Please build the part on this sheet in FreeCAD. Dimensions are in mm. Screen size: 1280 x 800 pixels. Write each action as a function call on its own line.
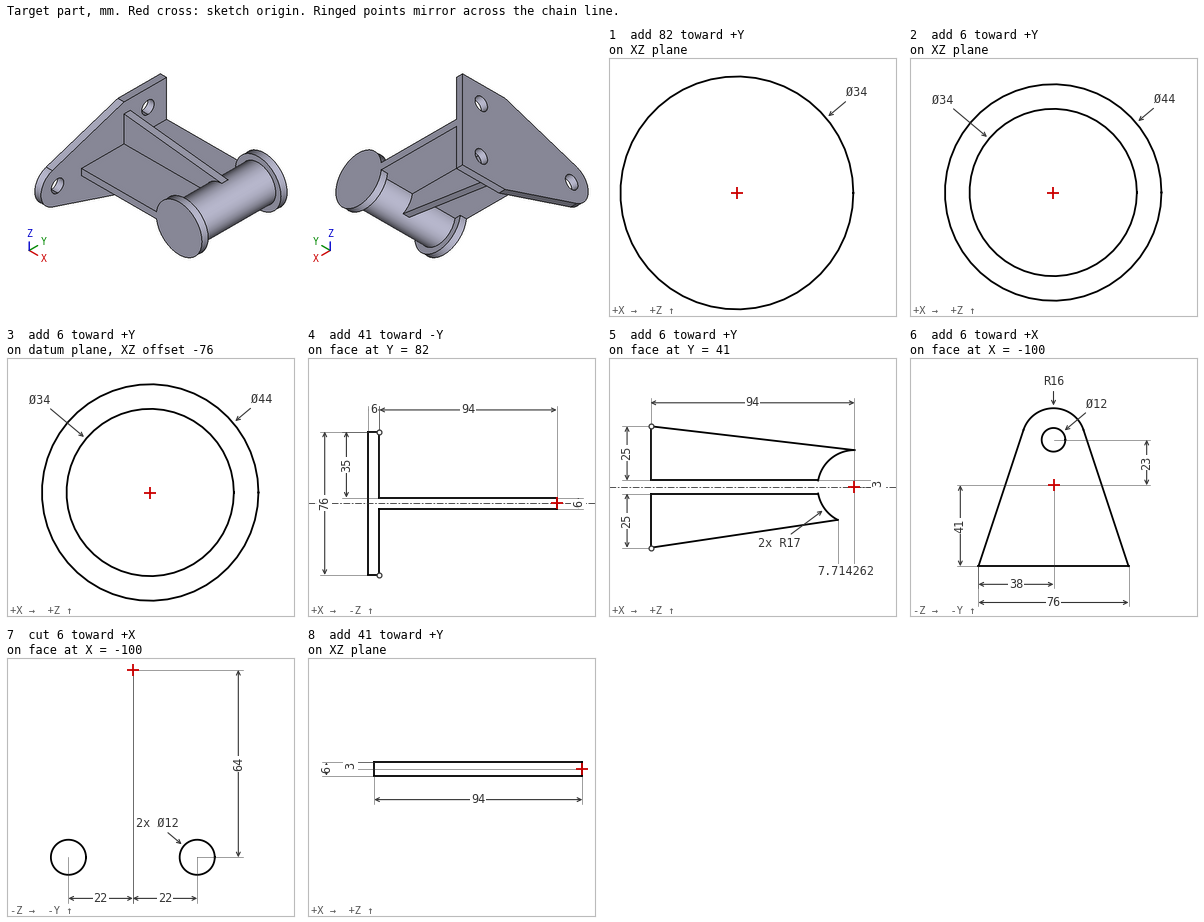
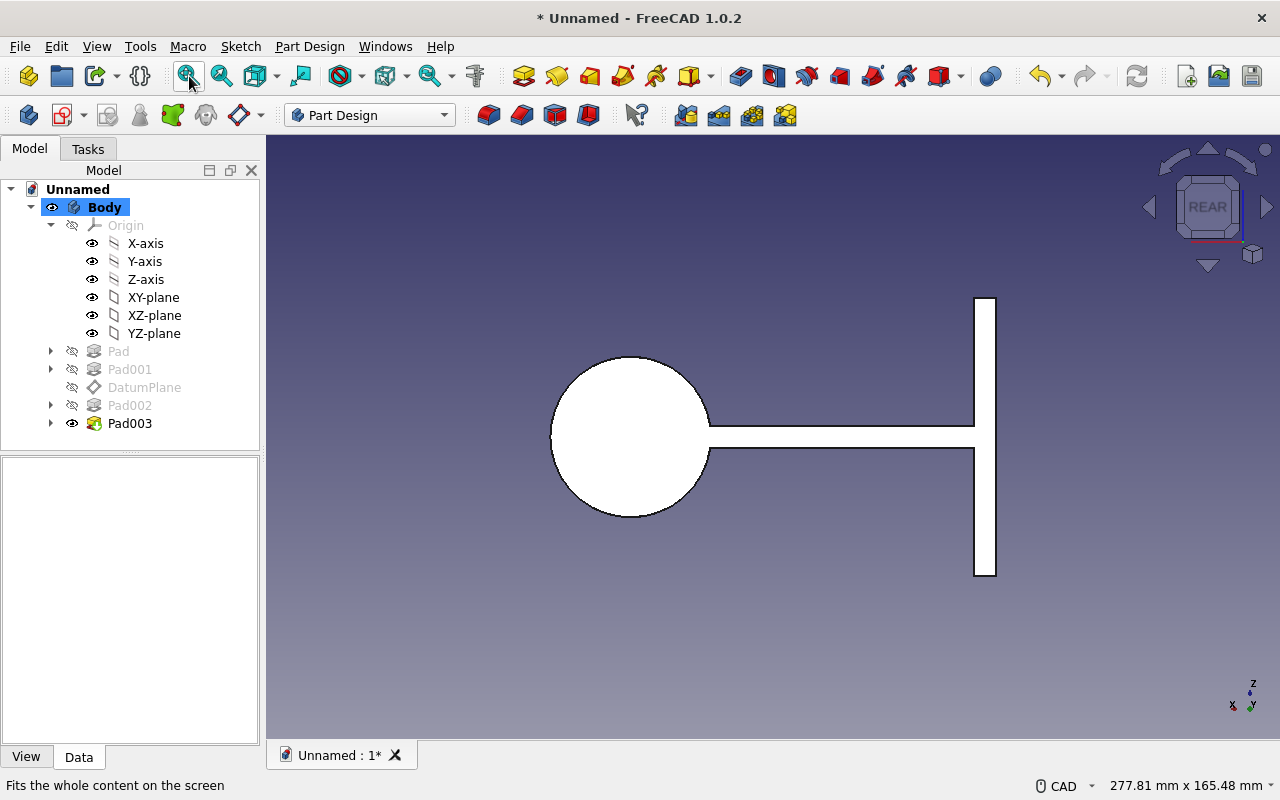
key(0)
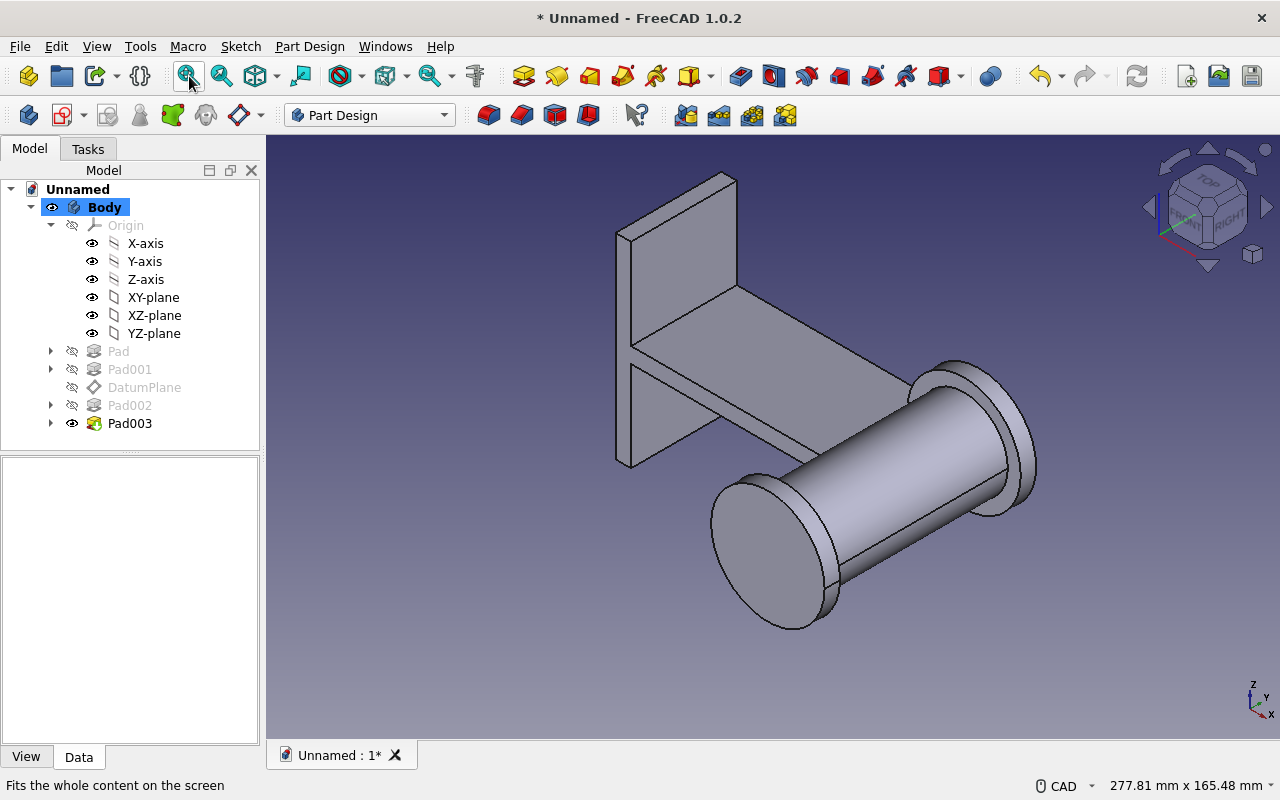
key(1)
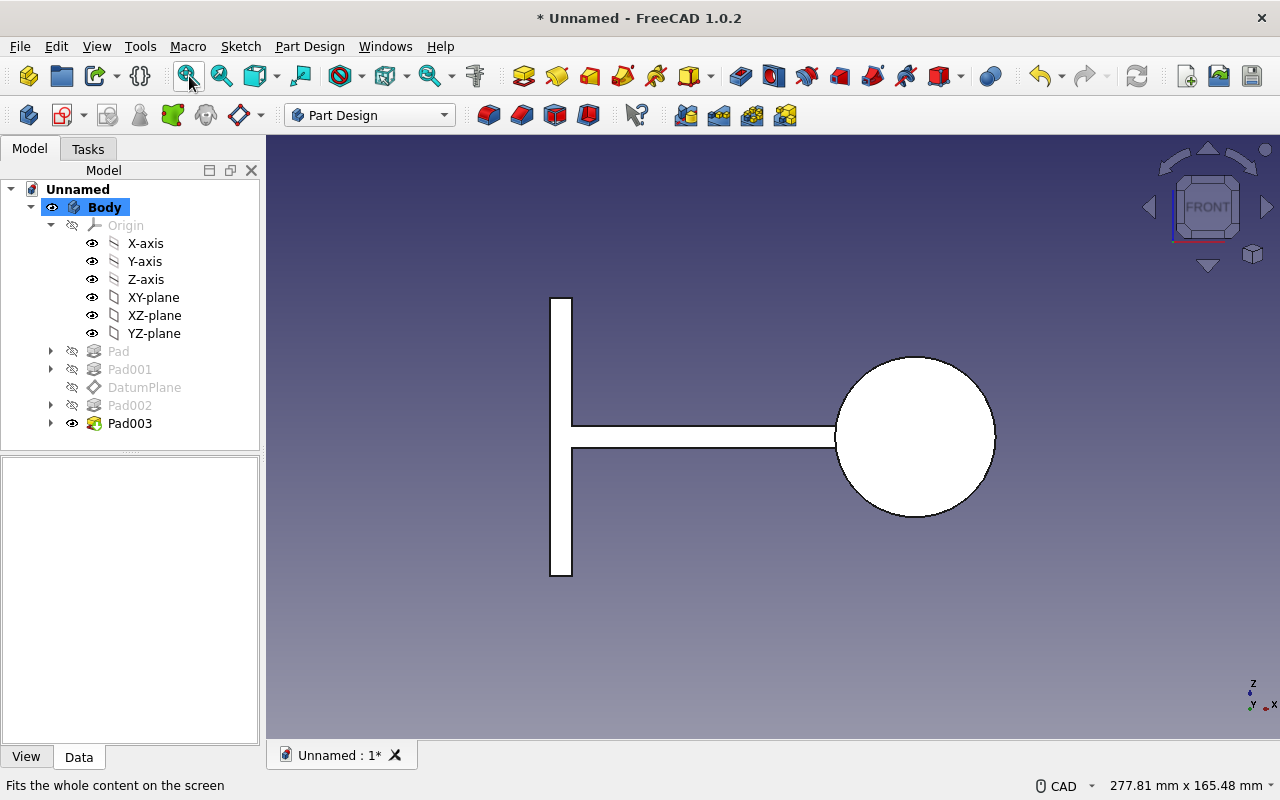
click(572, 436)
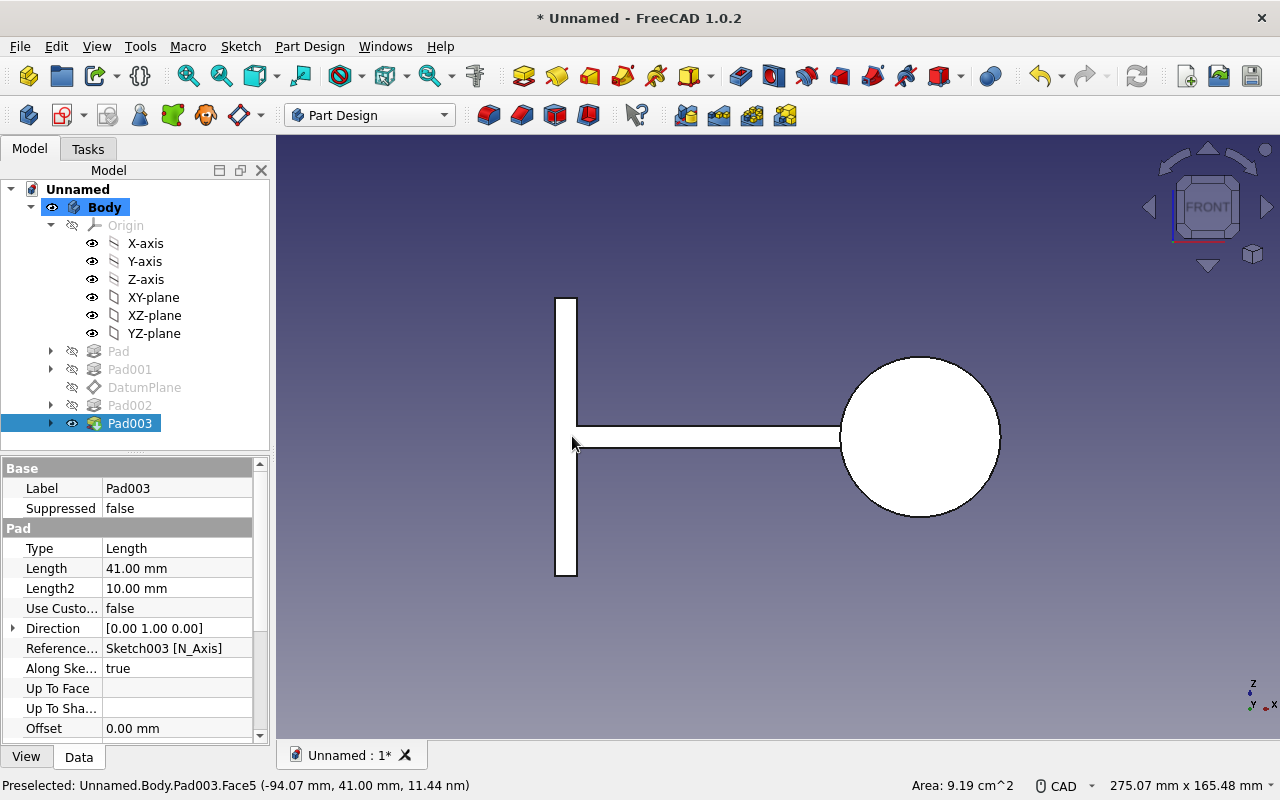
click(62, 116)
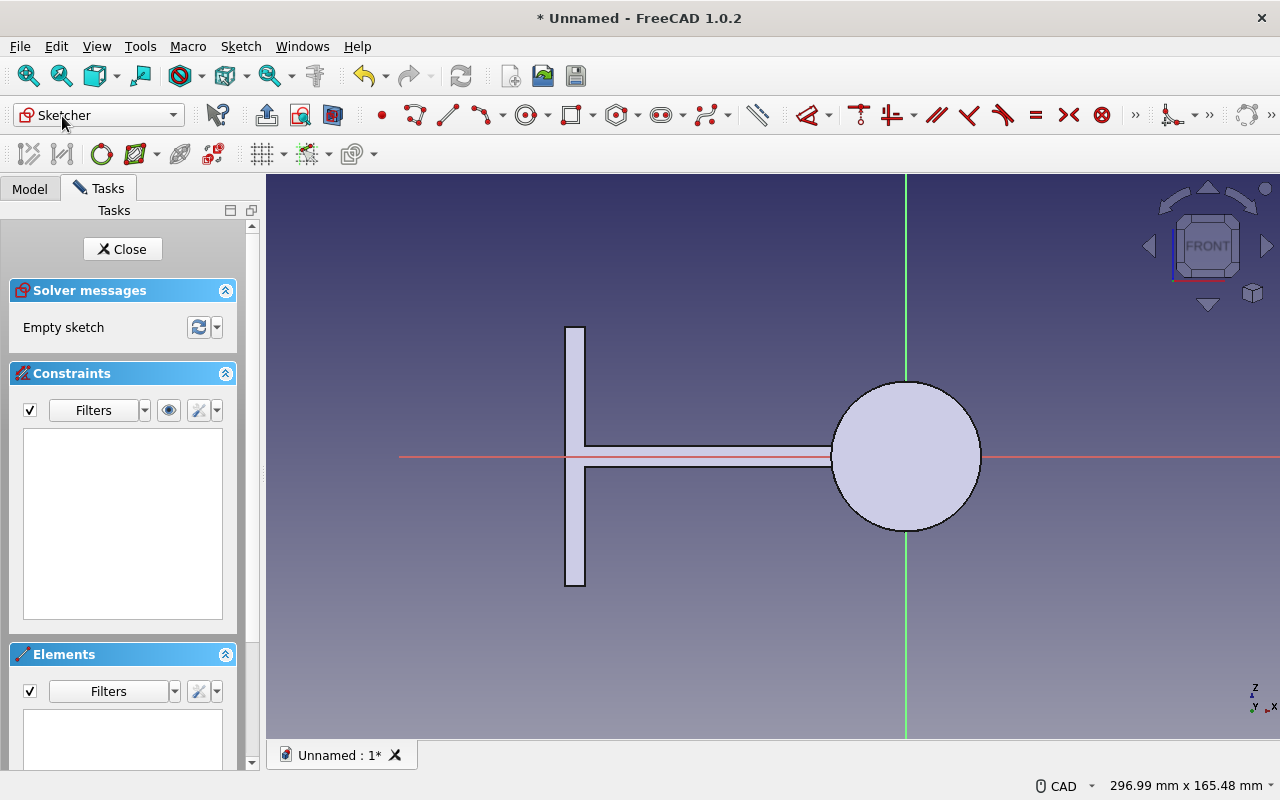
scroll(796, 457, up, 3)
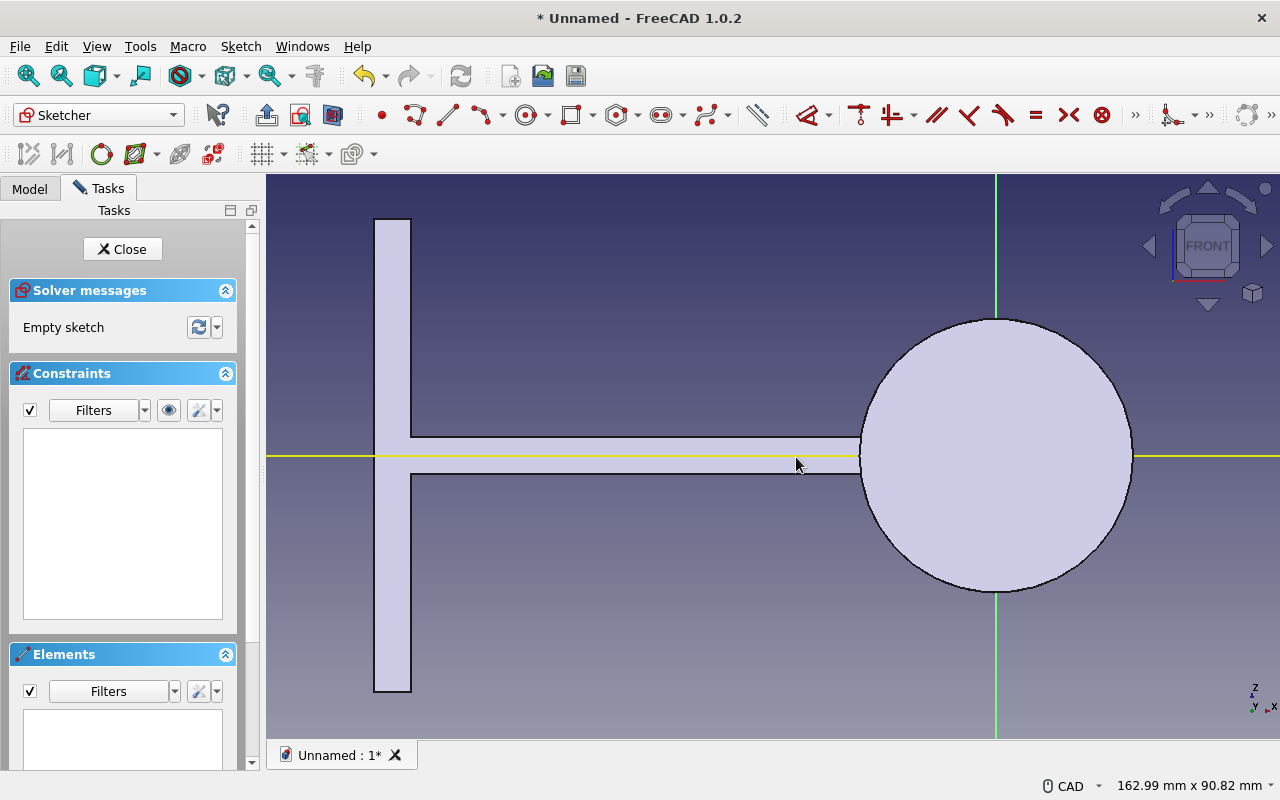
click(415, 116)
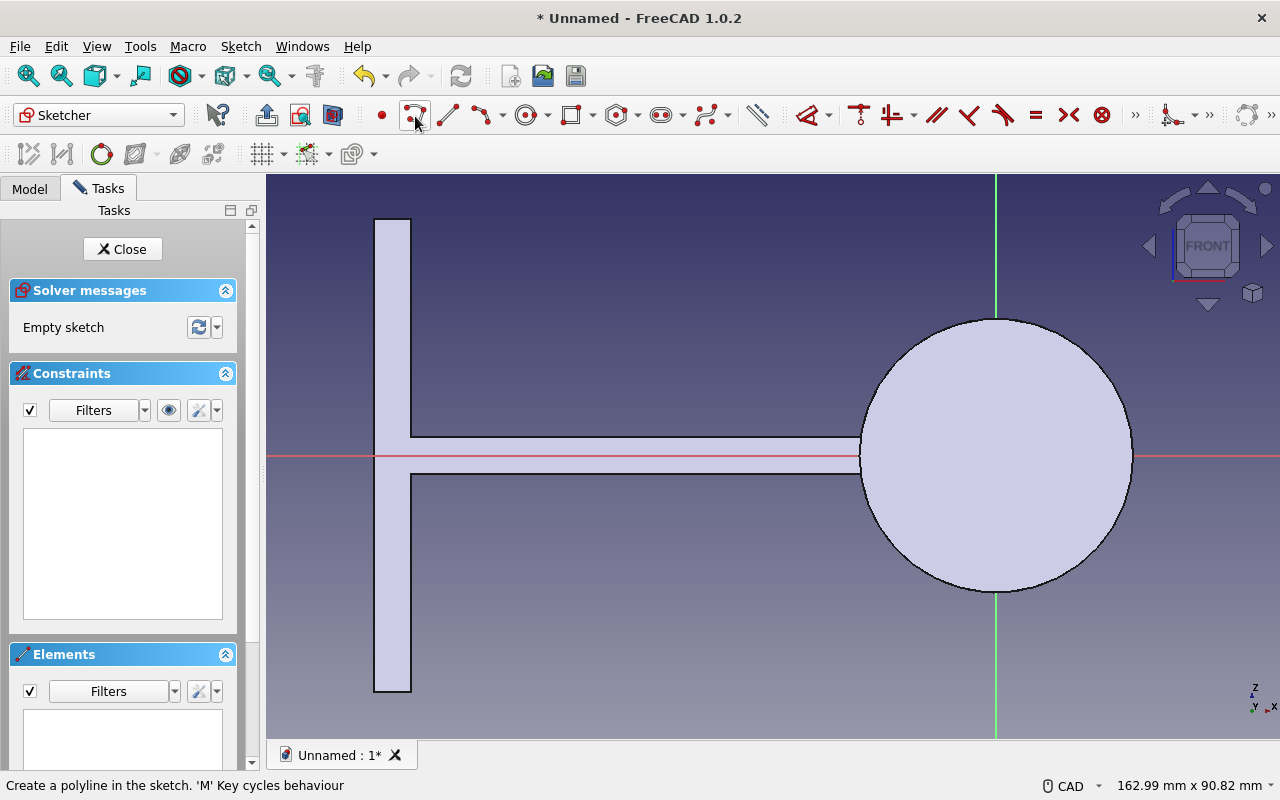
click(892, 437)
click(411, 437)
click(411, 281)
click(996, 350)
right_click(996, 350)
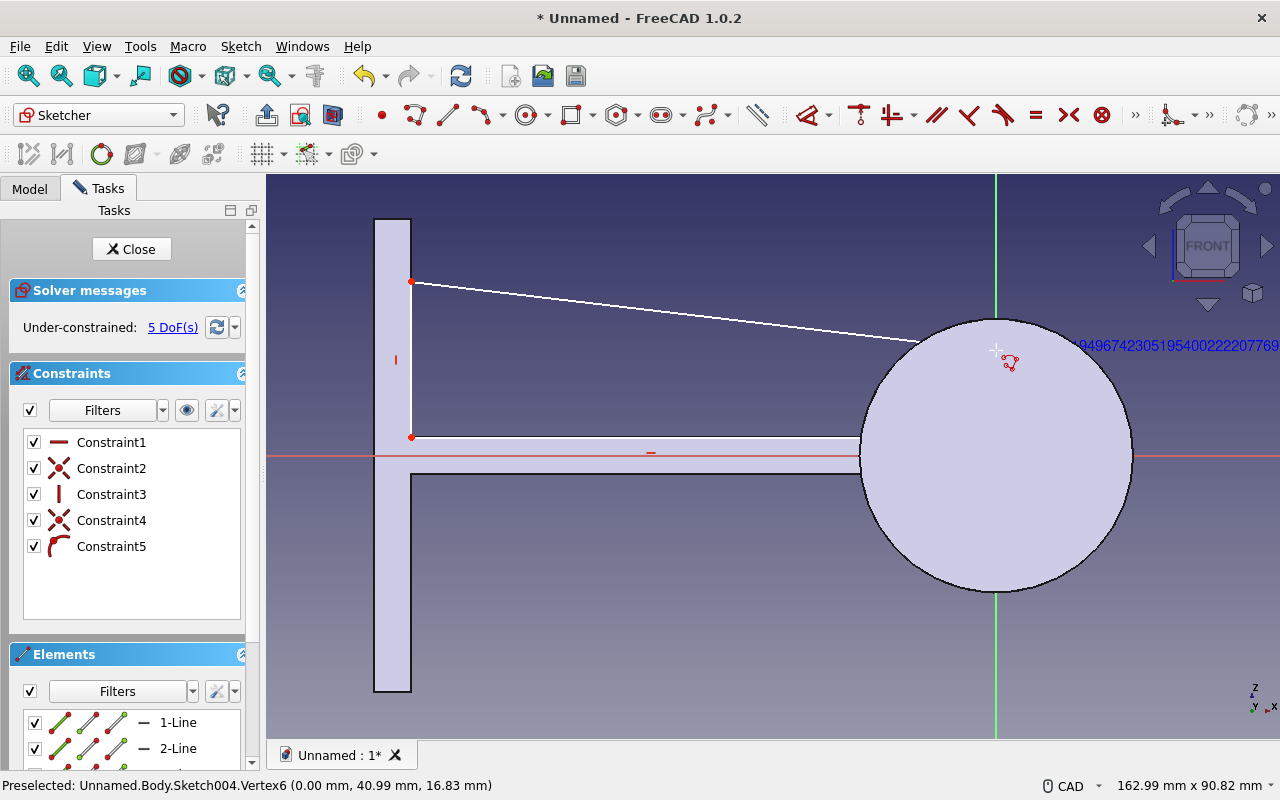
click(480, 116)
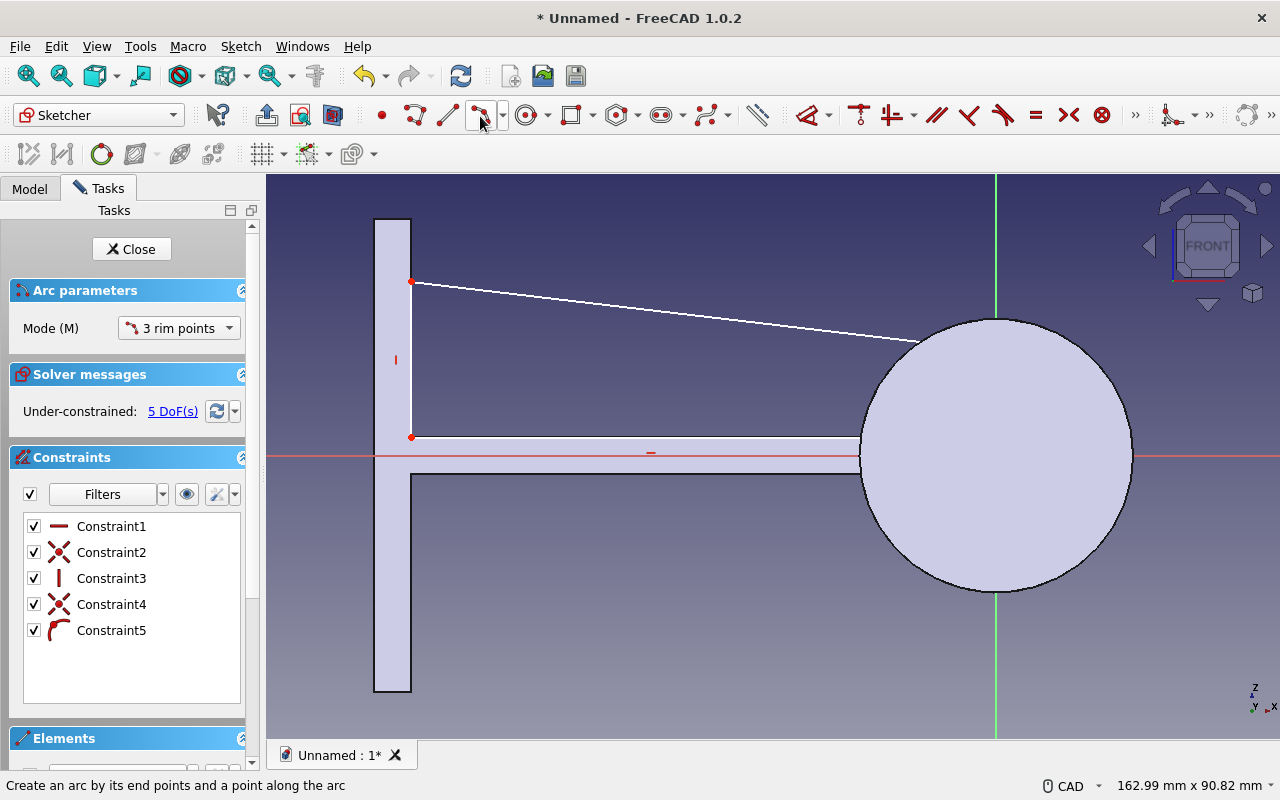
click(996, 351)
click(892, 438)
click(928, 375)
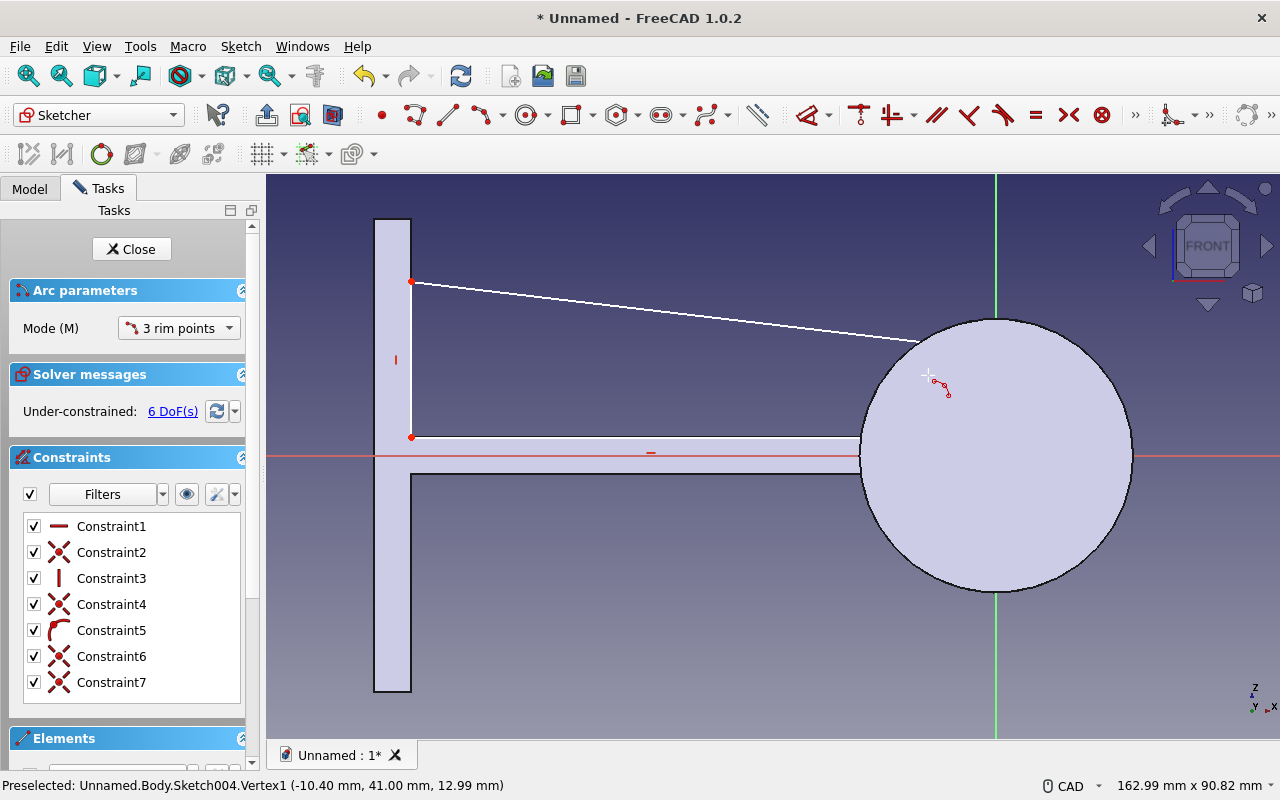
click(415, 116)